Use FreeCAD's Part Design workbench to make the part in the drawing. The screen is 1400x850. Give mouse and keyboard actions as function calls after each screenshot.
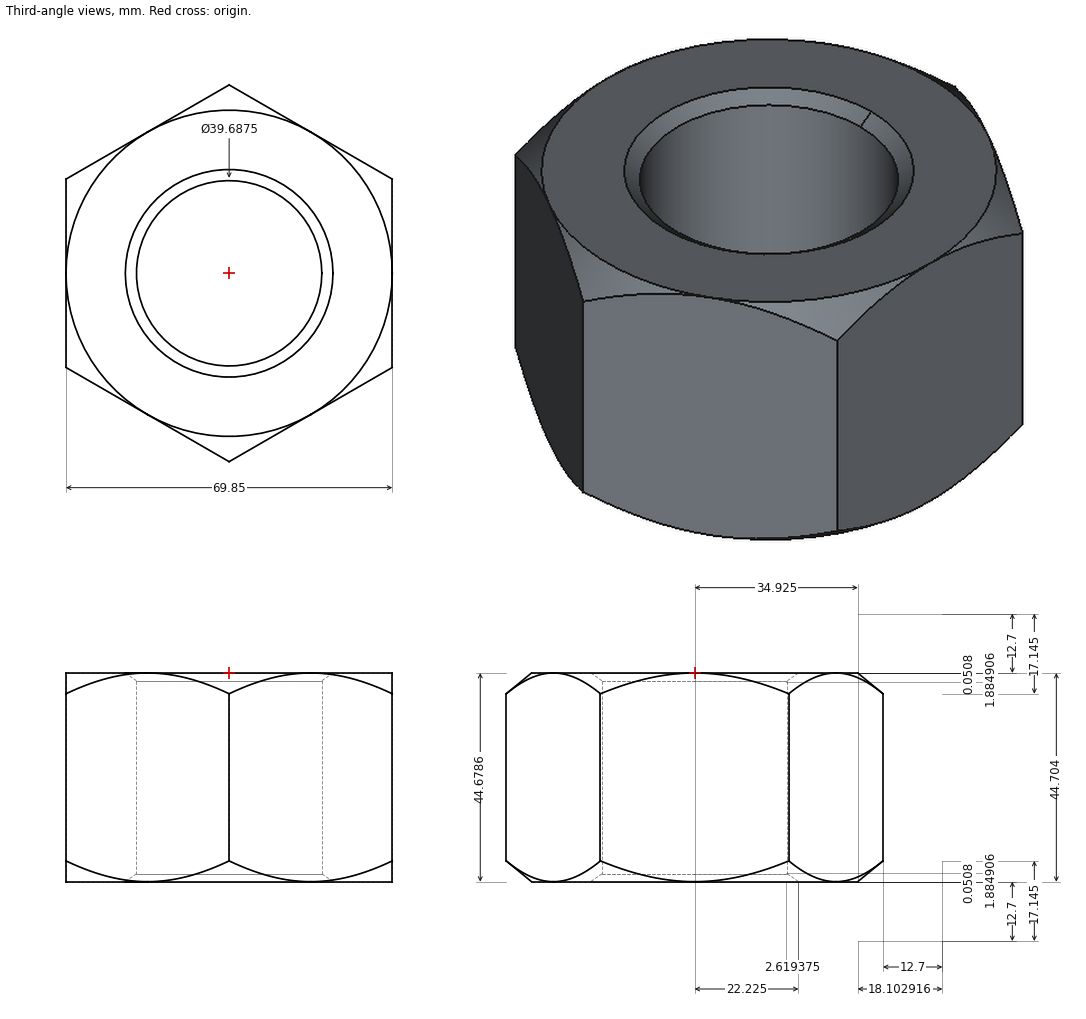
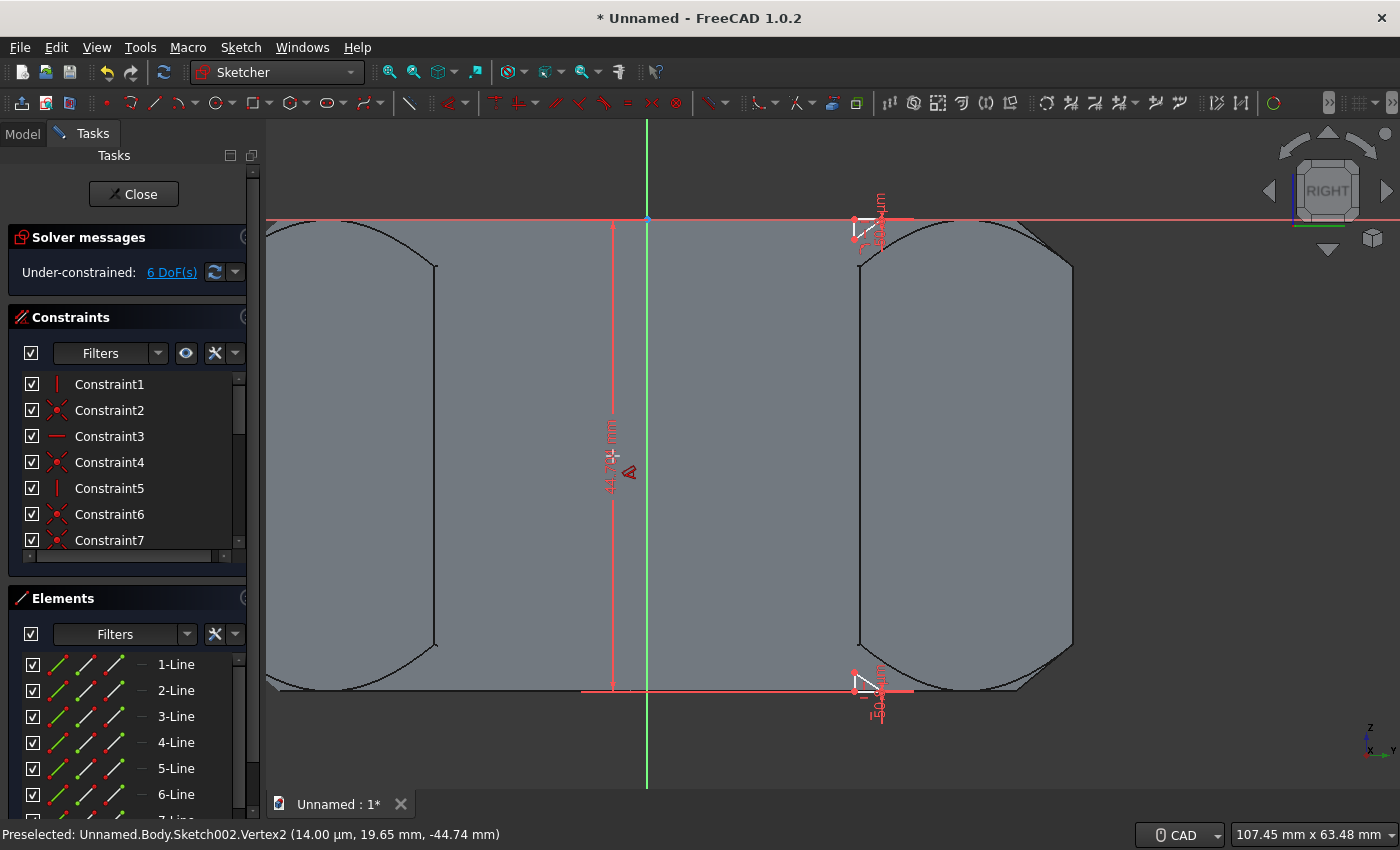
scroll(882, 692, up, 14)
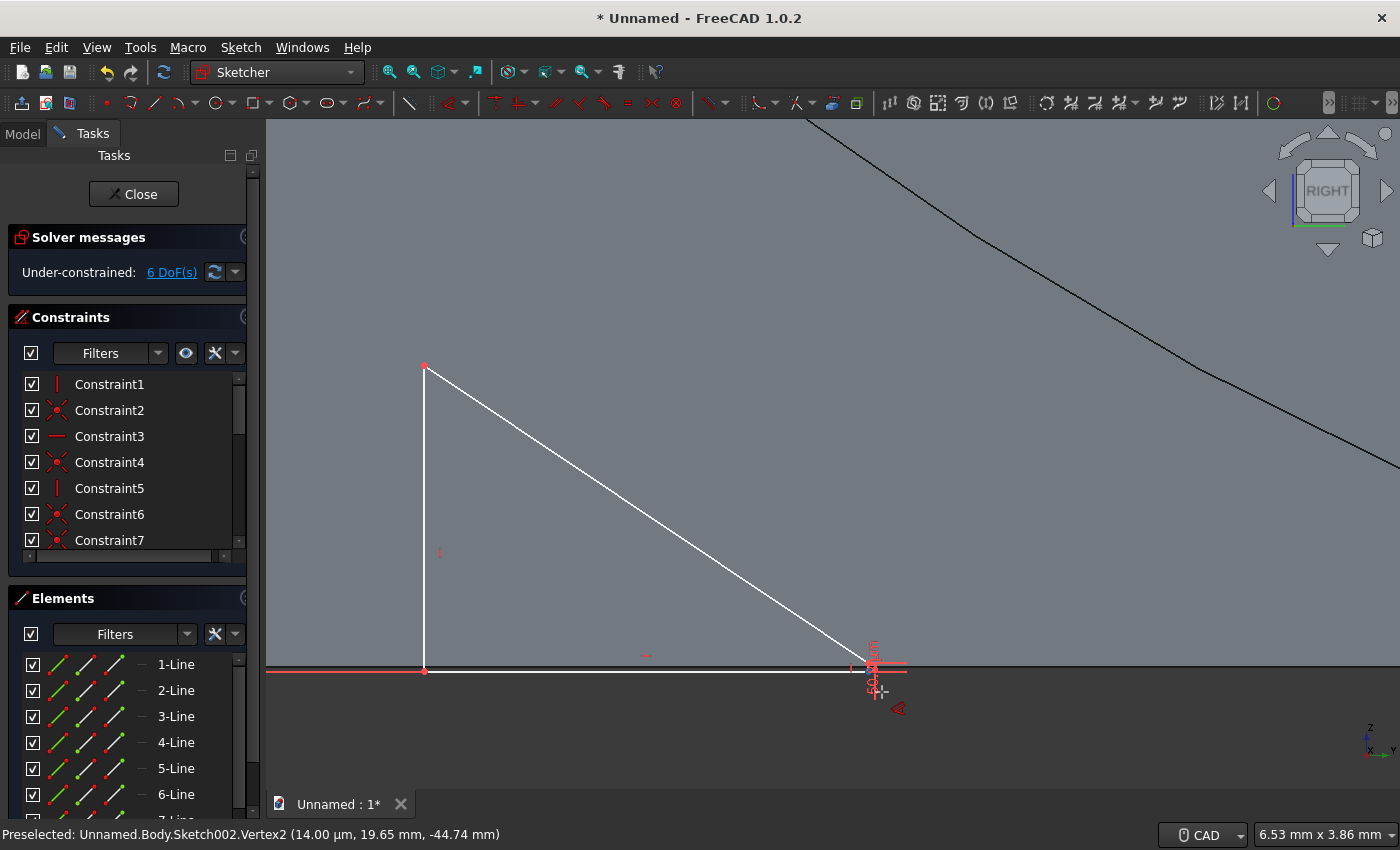
click(868, 672)
click(581, 706)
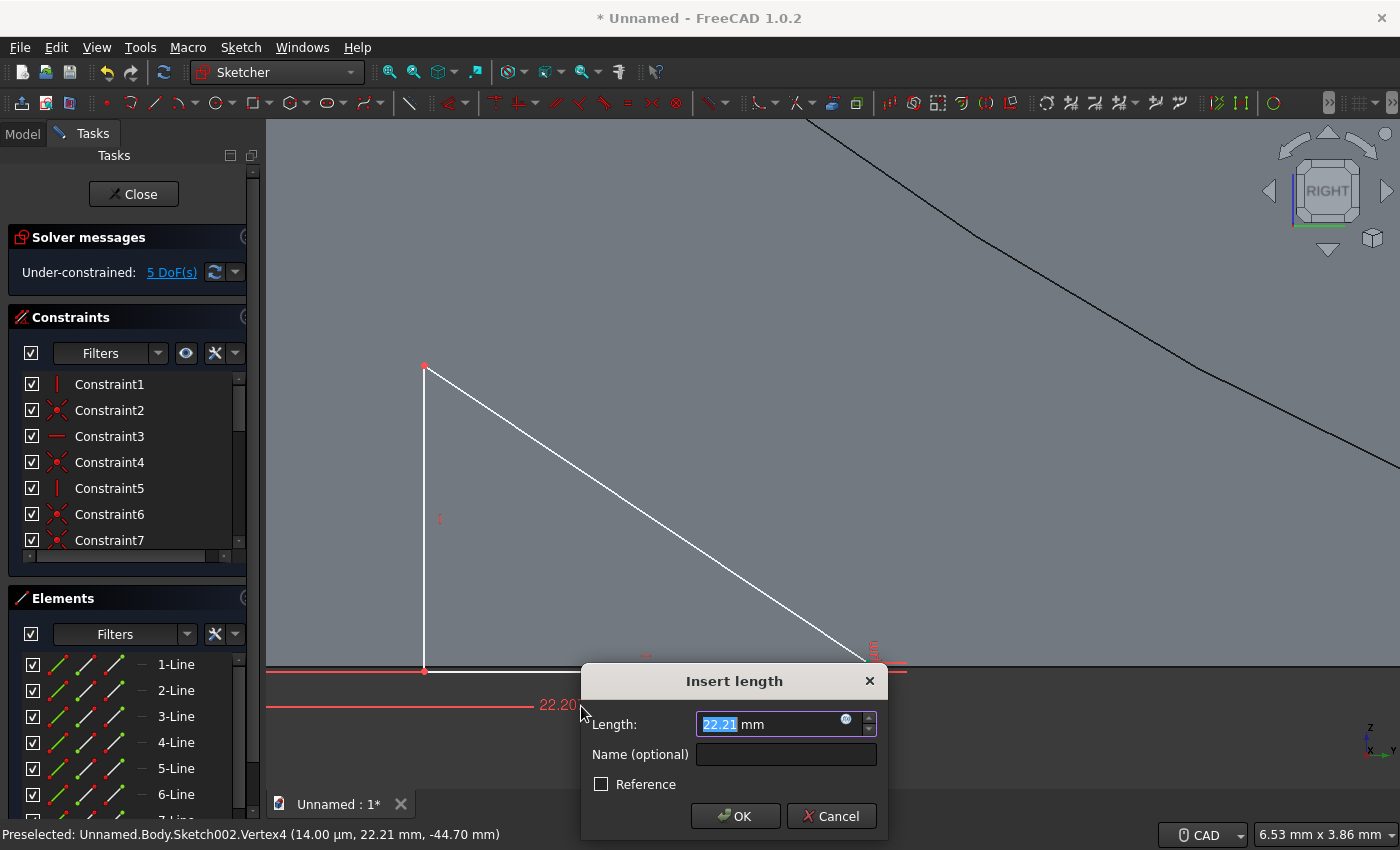
text(22.225)
key(Return)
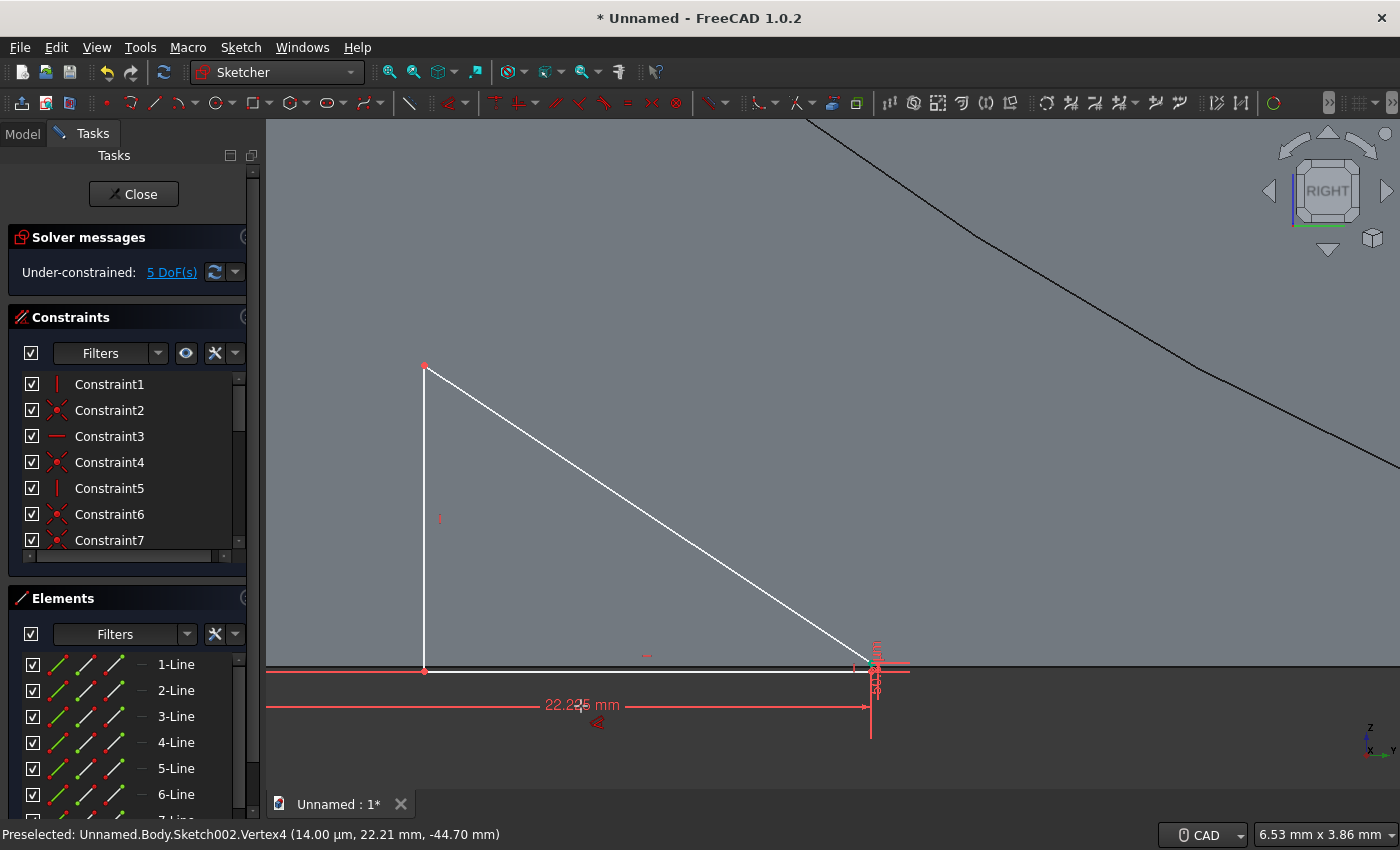
scroll(882, 691, down, 14)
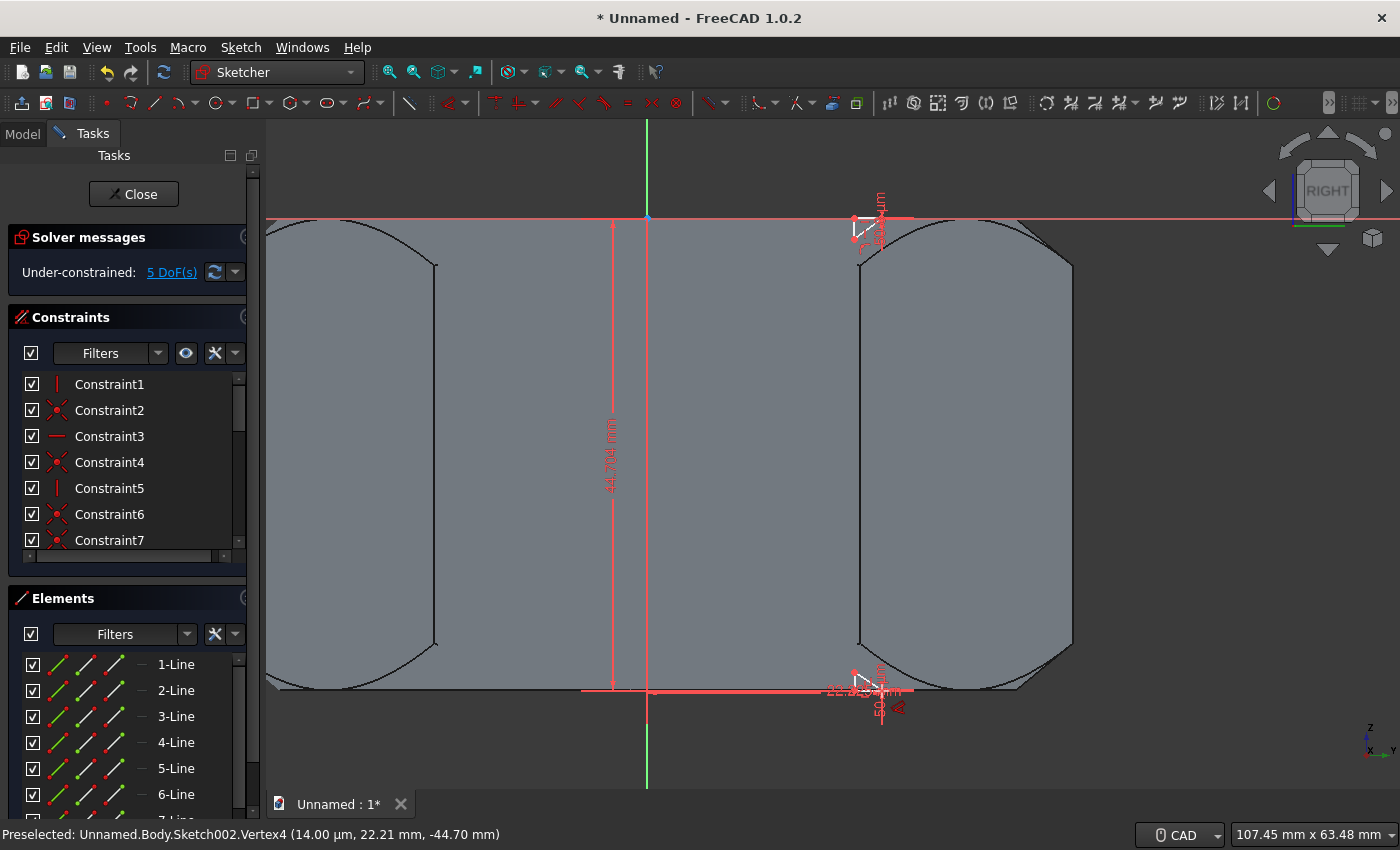
scroll(882, 219, up, 14)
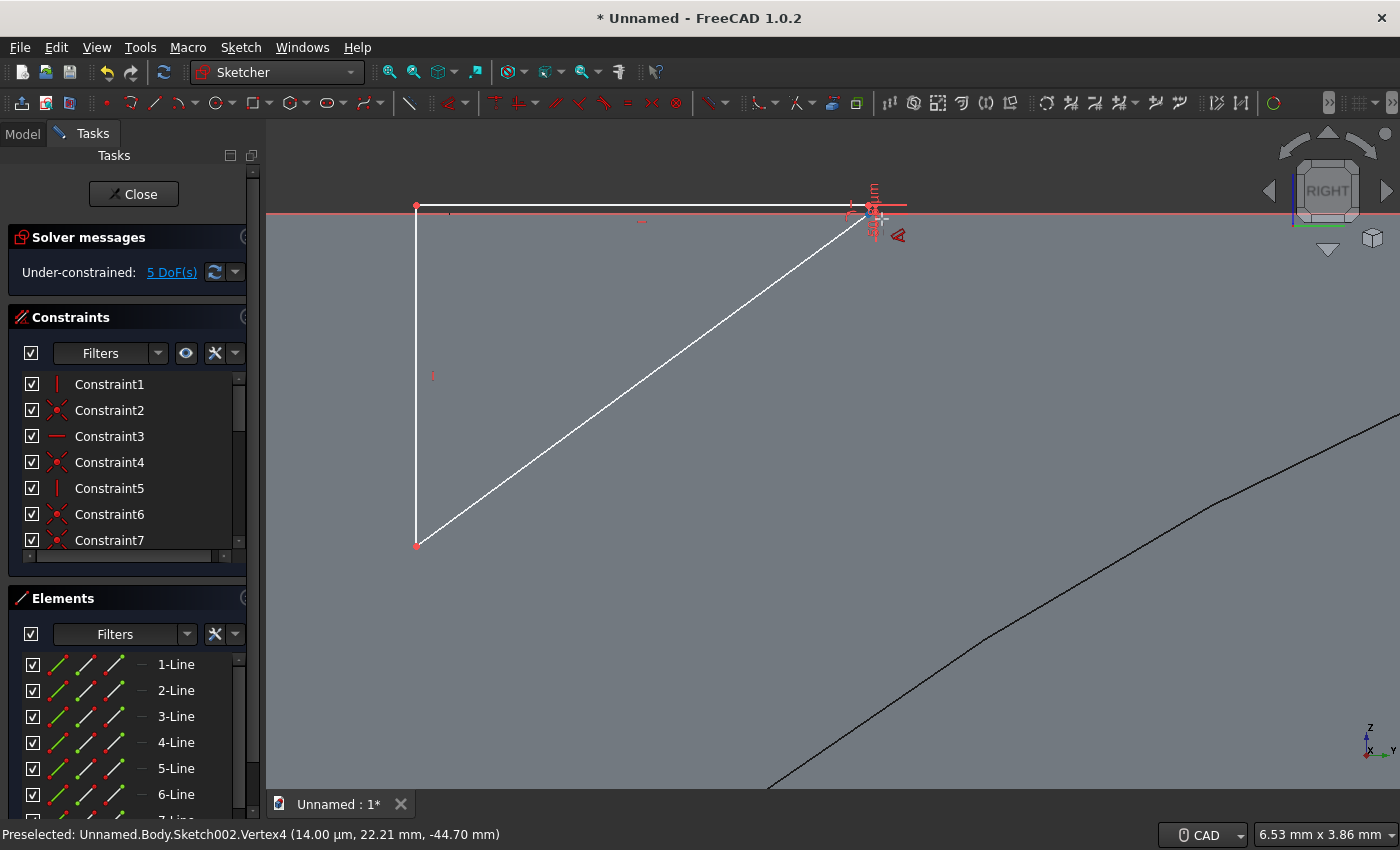
click(869, 214)
click(581, 180)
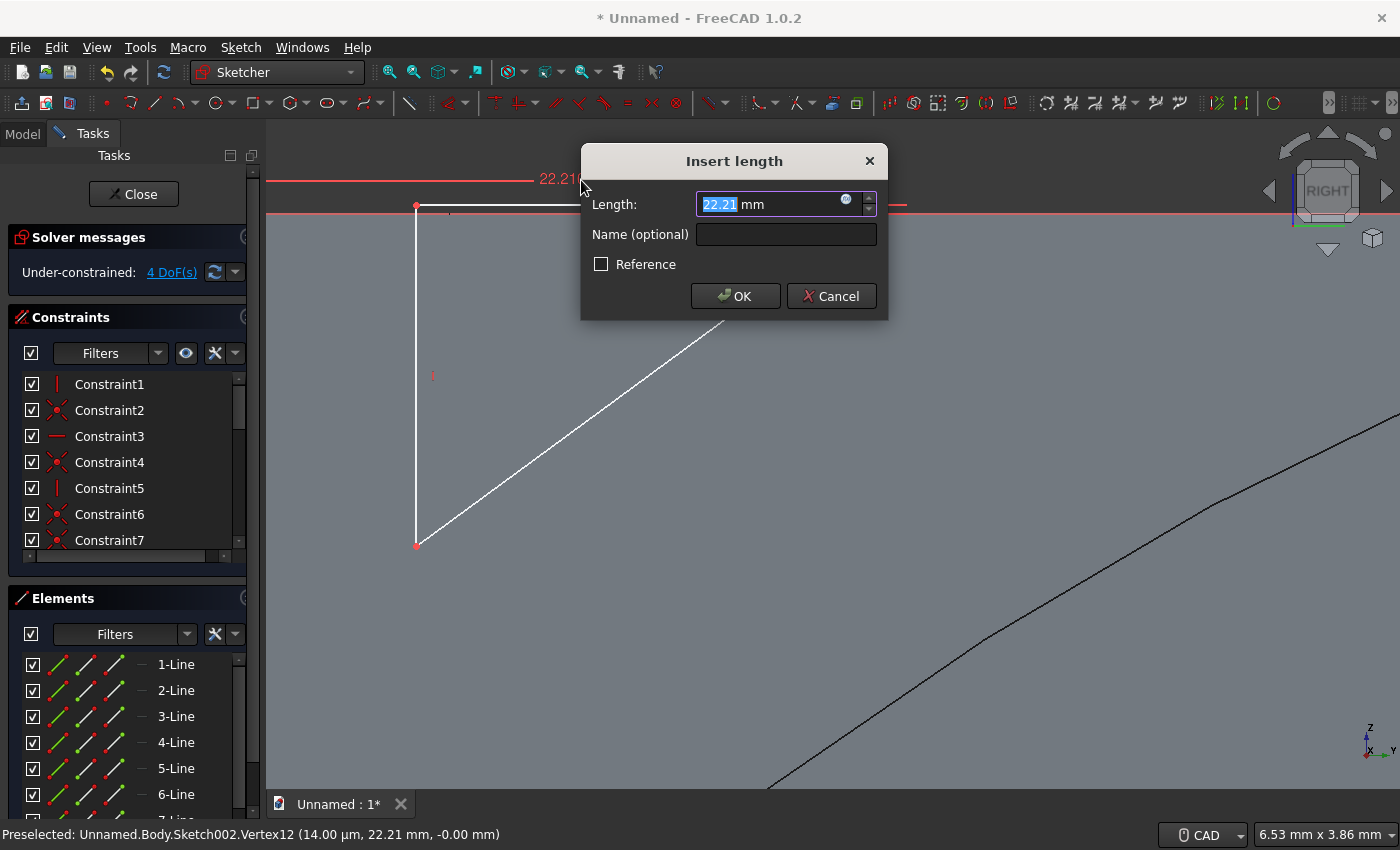
text(22.225)
key(Return)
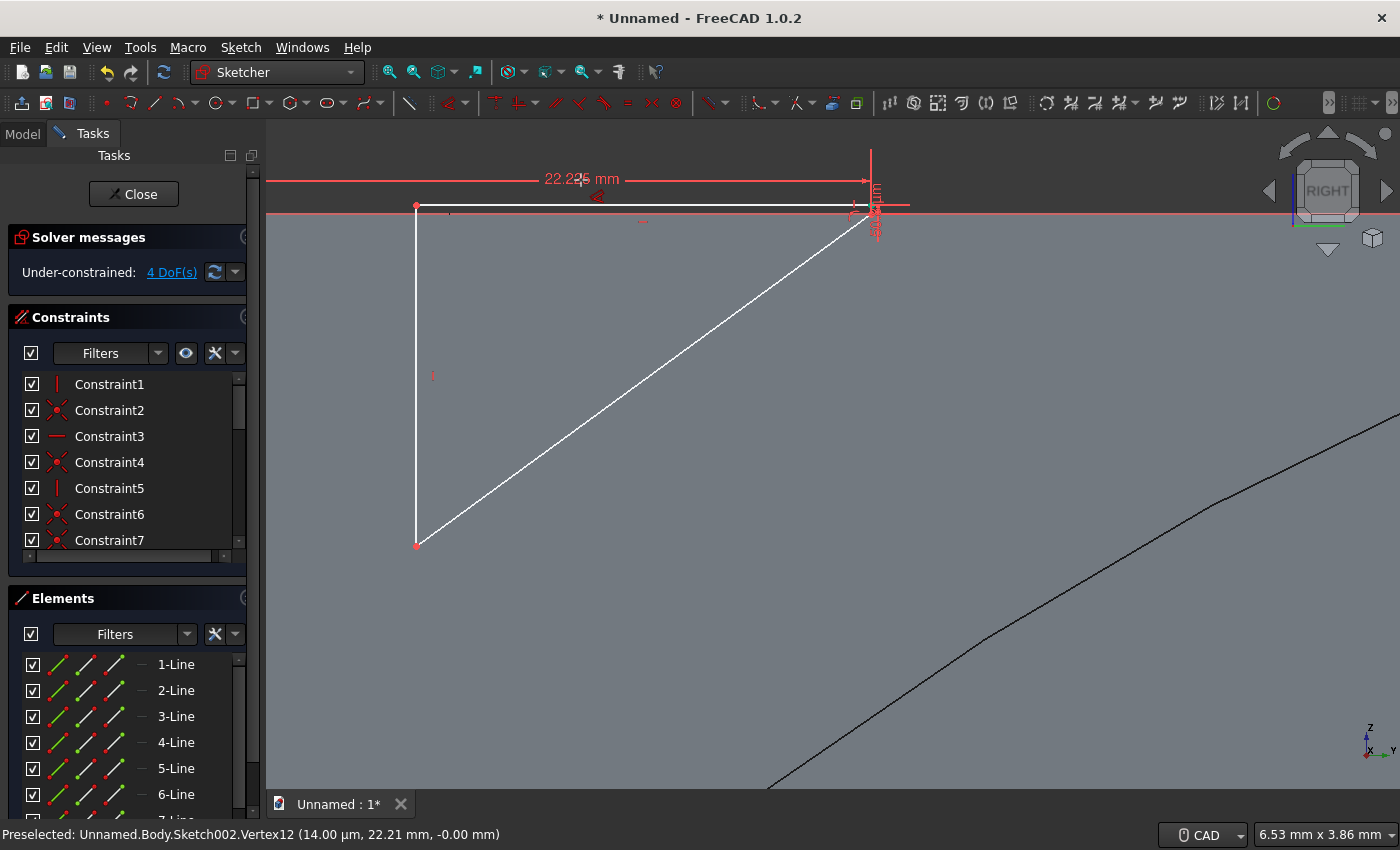
scroll(882, 219, down, 14)